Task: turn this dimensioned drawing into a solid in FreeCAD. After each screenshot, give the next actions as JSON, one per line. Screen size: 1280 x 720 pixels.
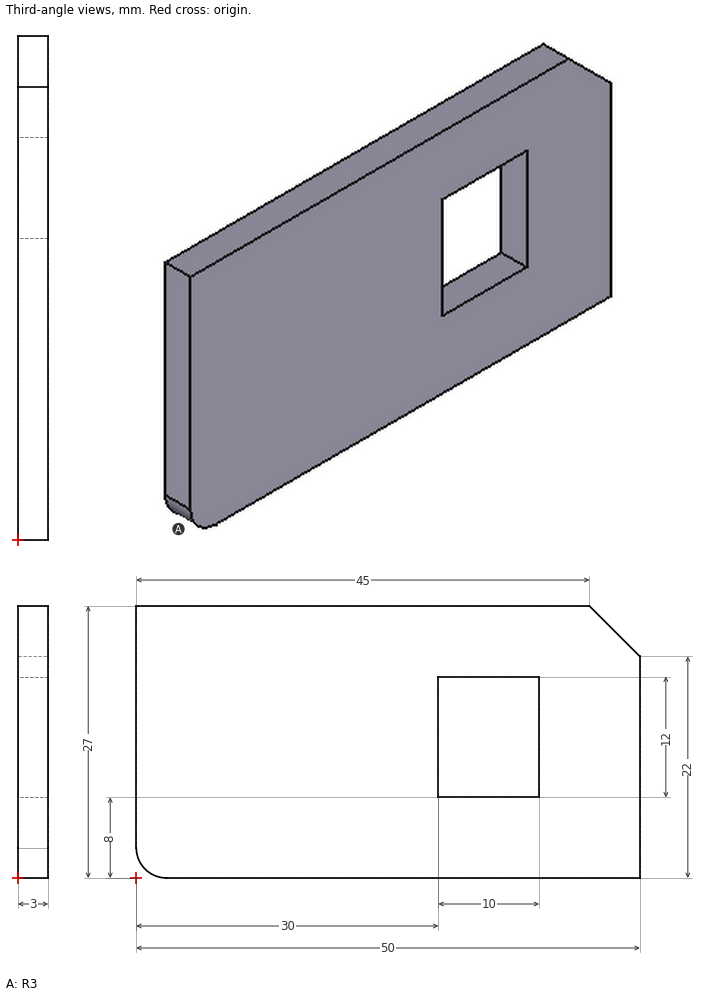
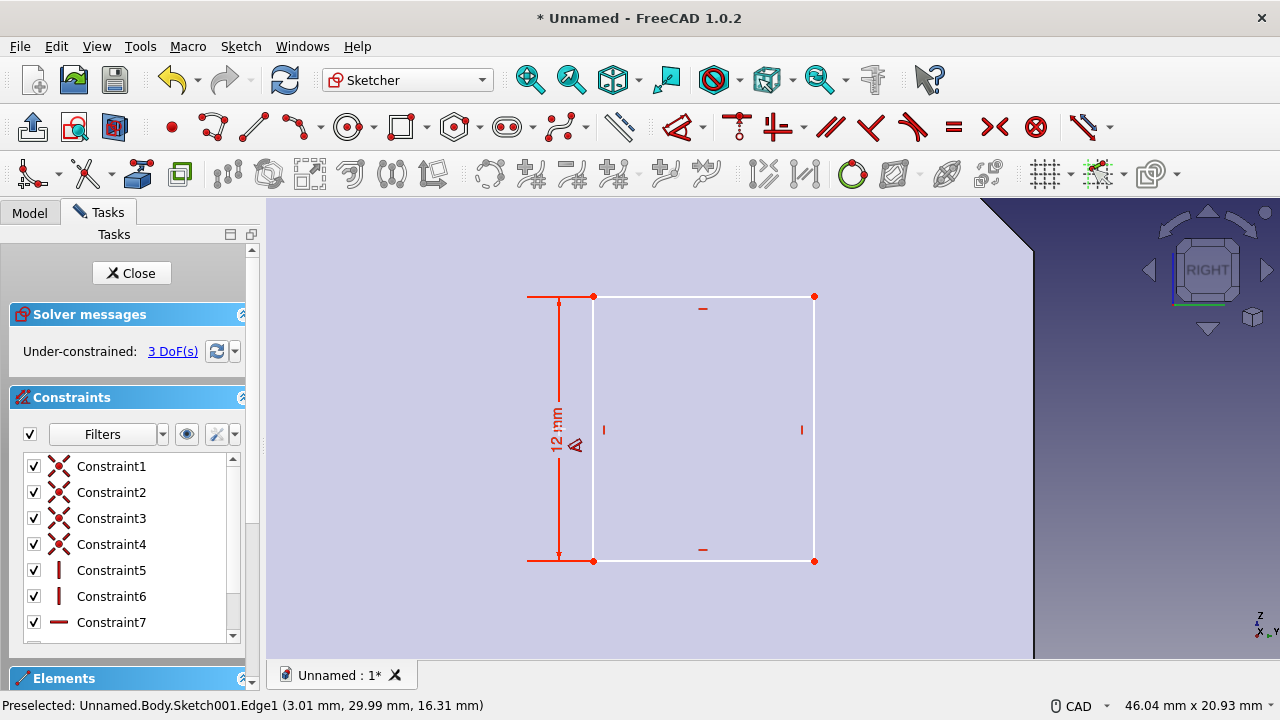
{"action": "left_click", "coordinate": [659, 561]}
{"action": "left_click", "coordinate": [704, 595]}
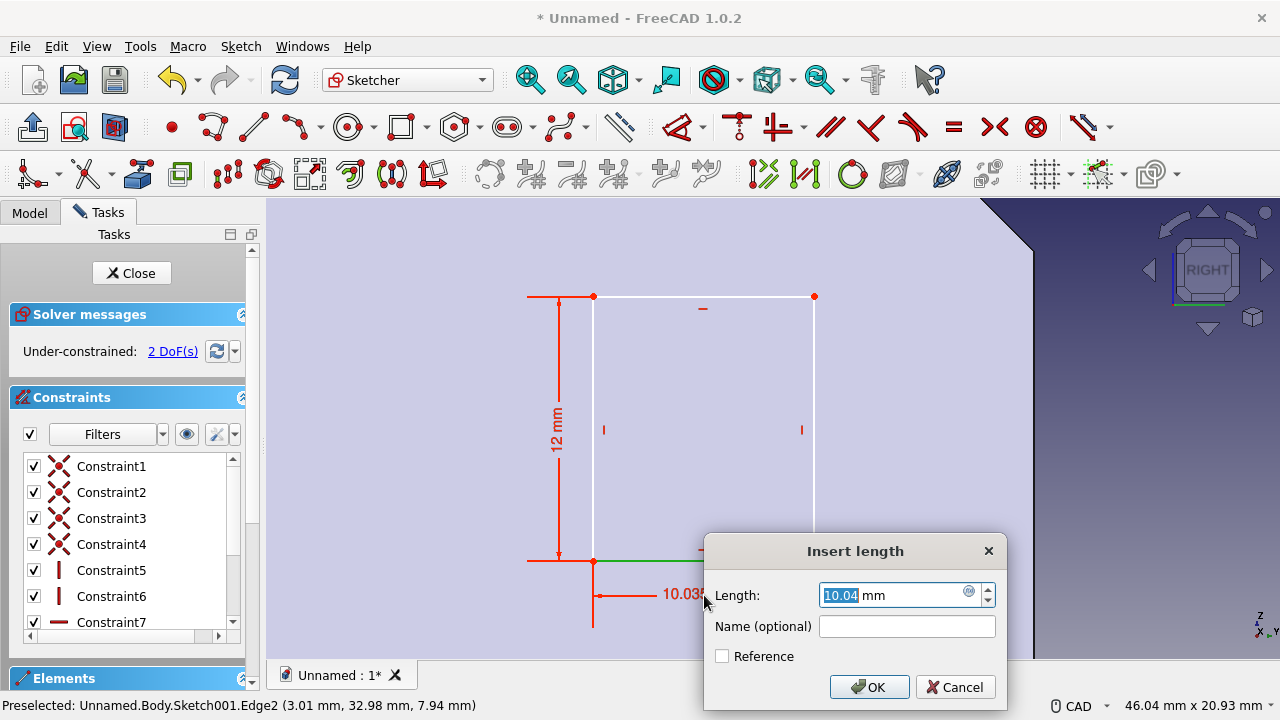
{"action": "type", "text": "10"}
{"action": "key", "text": "Return"}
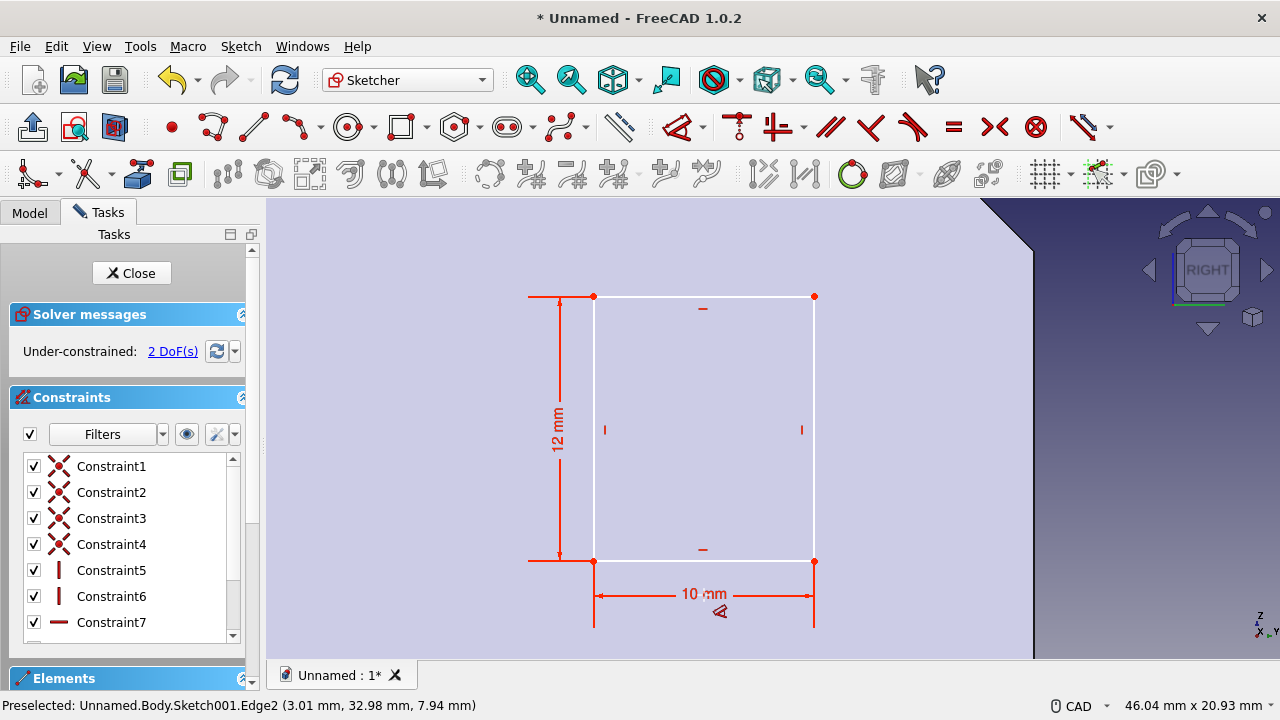
{"action": "left_click", "coordinate": [594, 561]}
{"action": "left_click", "coordinate": [628, 596]}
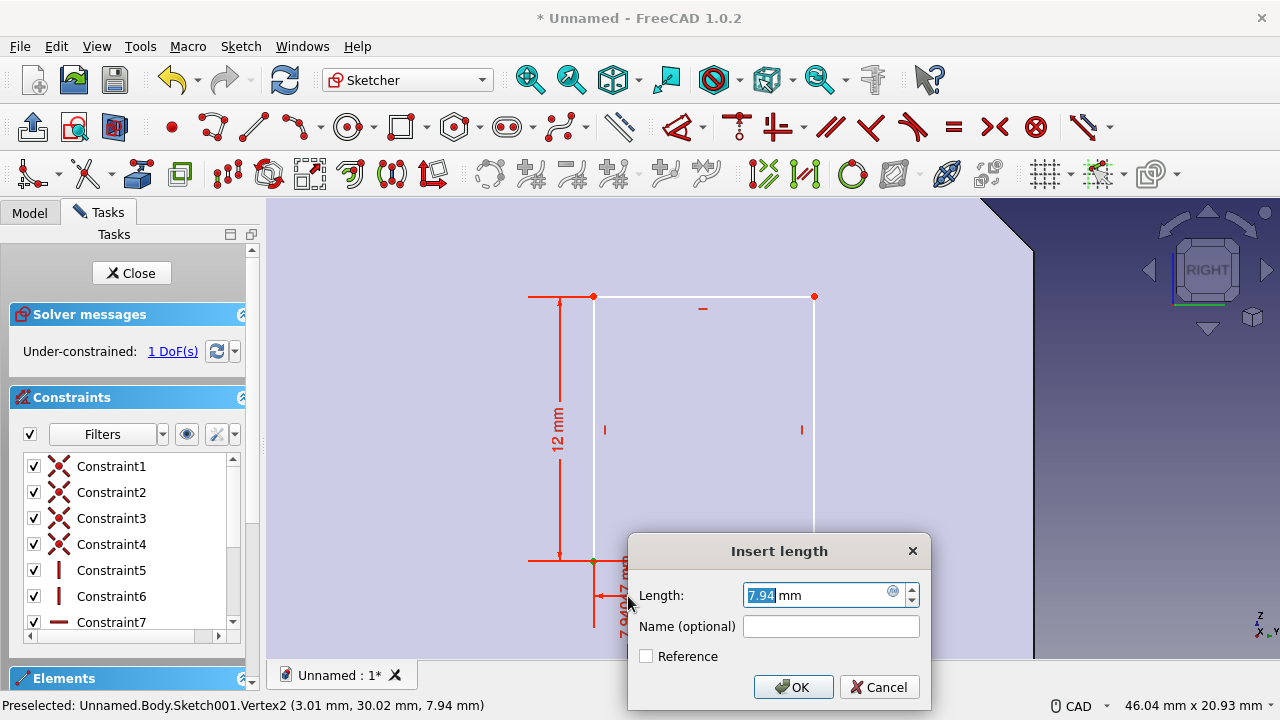
{"action": "type", "text": "8"}
{"action": "key", "text": "Return"}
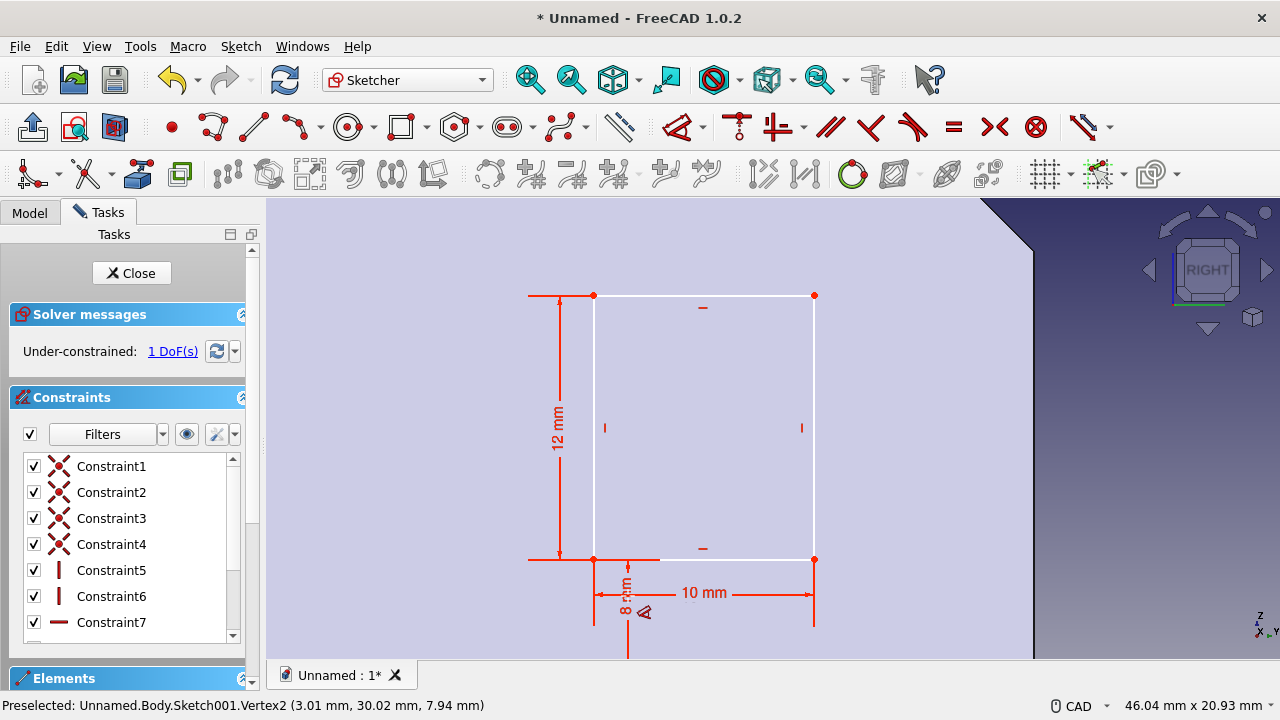
{"action": "left_click", "coordinate": [594, 296]}
{"action": "left_click", "coordinate": [444, 262]}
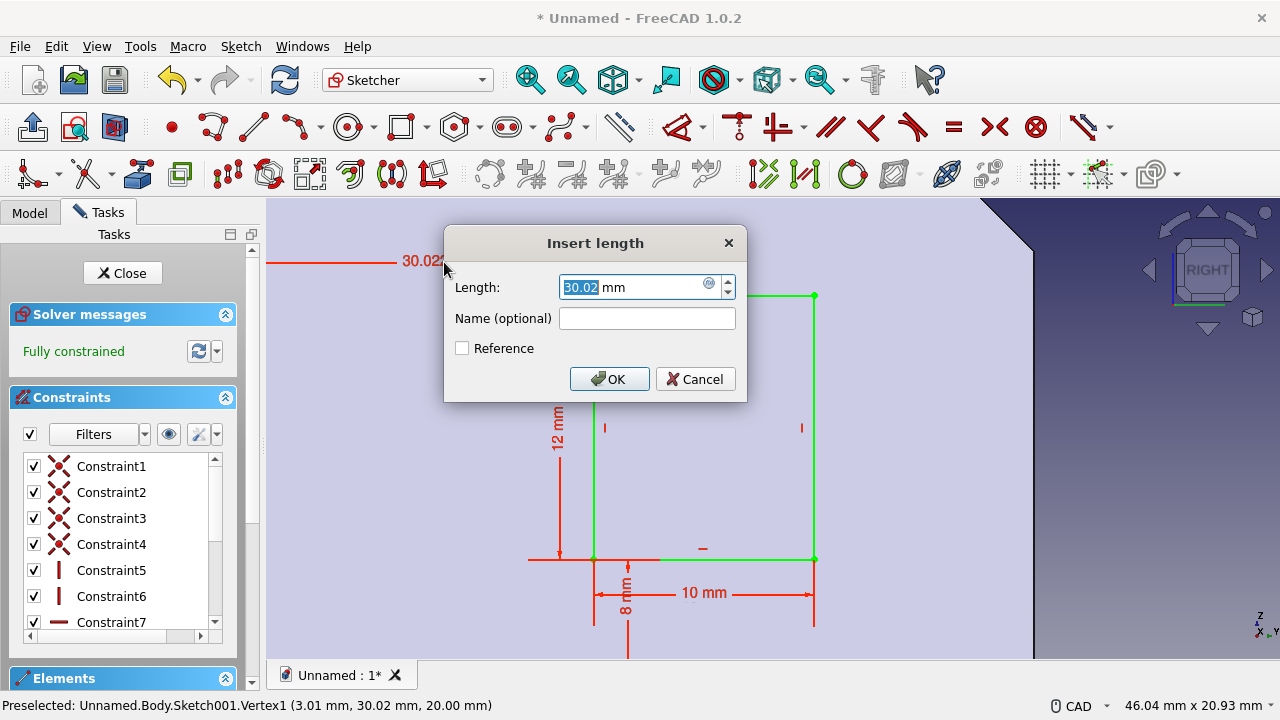
{"action": "type", "text": "30"}
{"action": "key", "text": "Return"}
{"action": "key", "text": "Escape"}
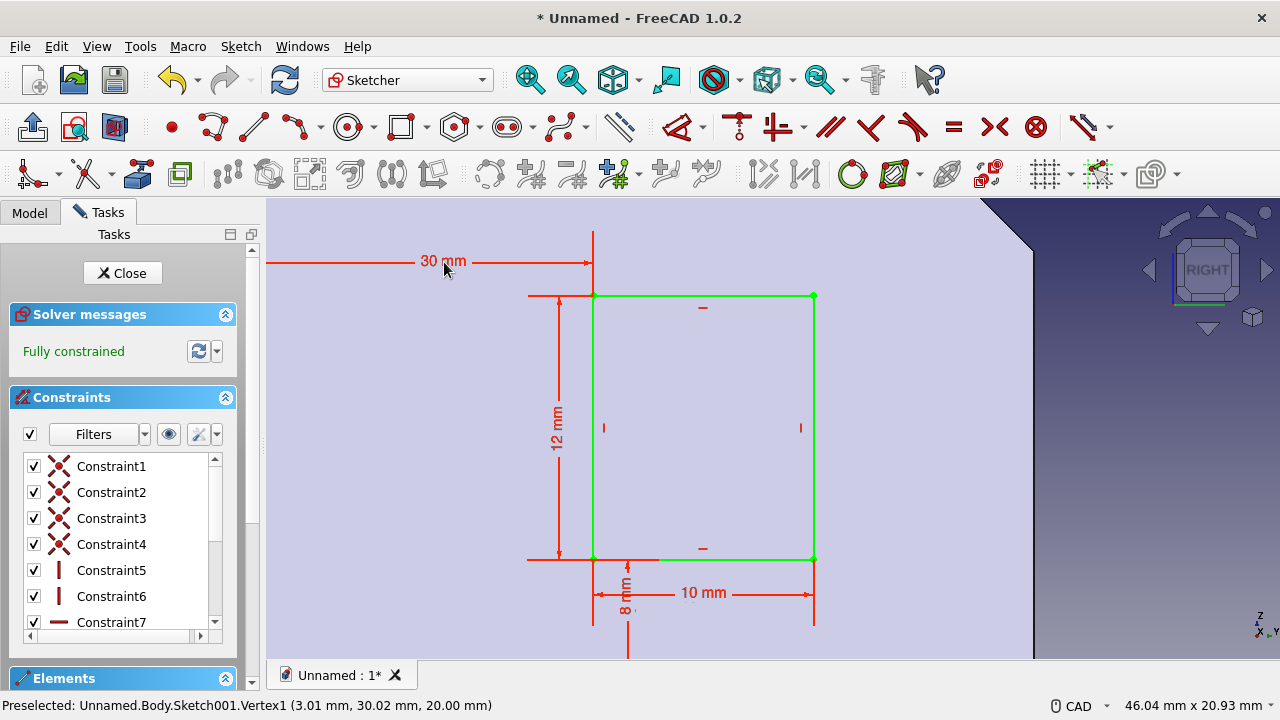
{"action": "left_click", "coordinate": [123, 273]}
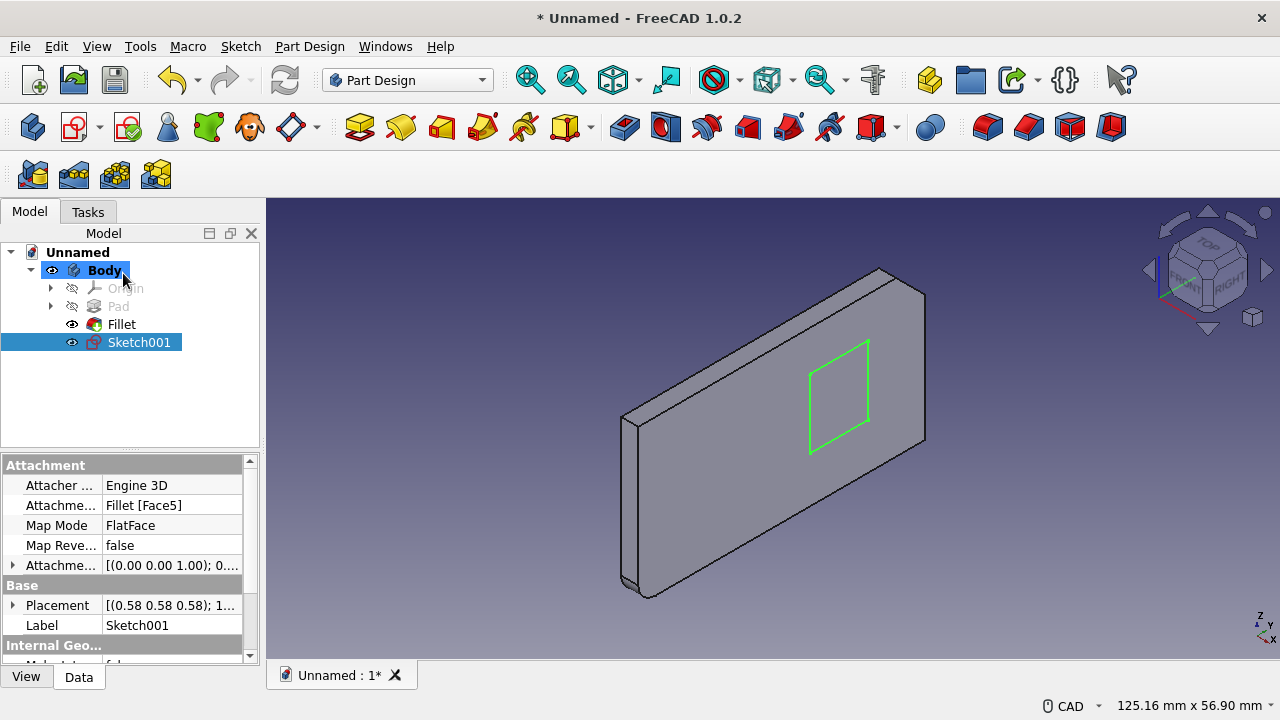
{"action": "left_click", "coordinate": [625, 128]}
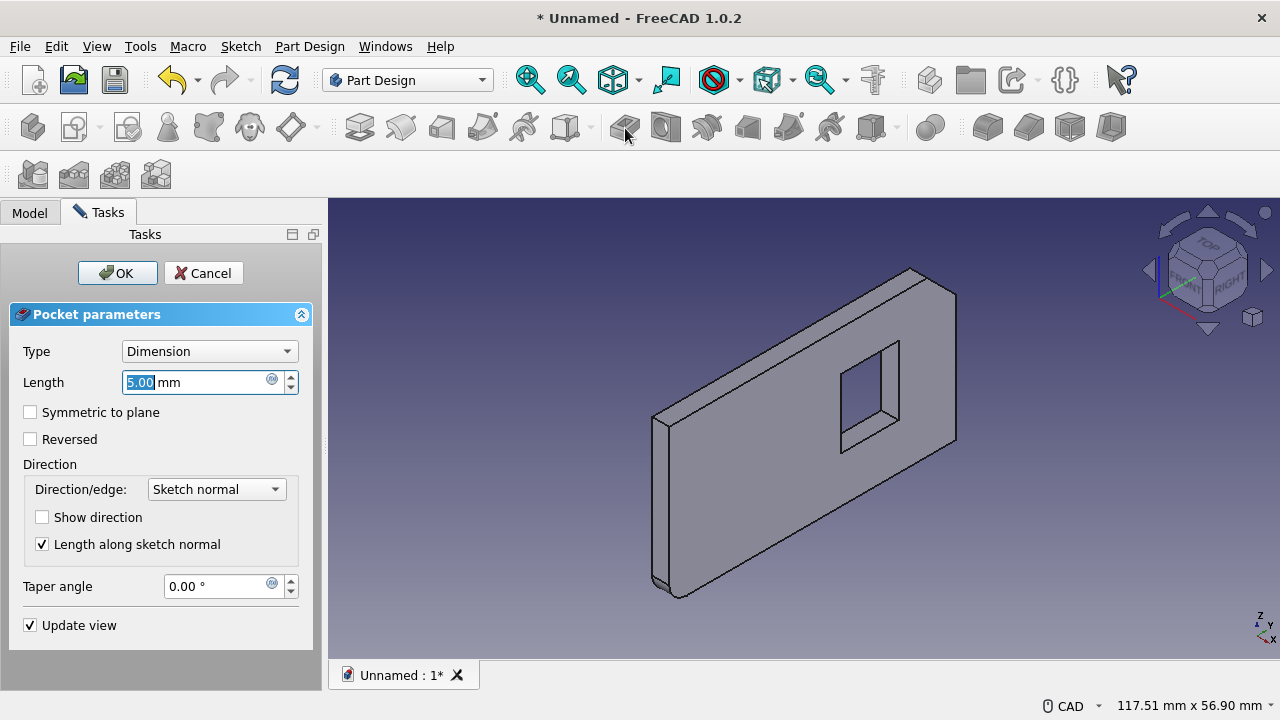
{"action": "left_click", "coordinate": [210, 352]}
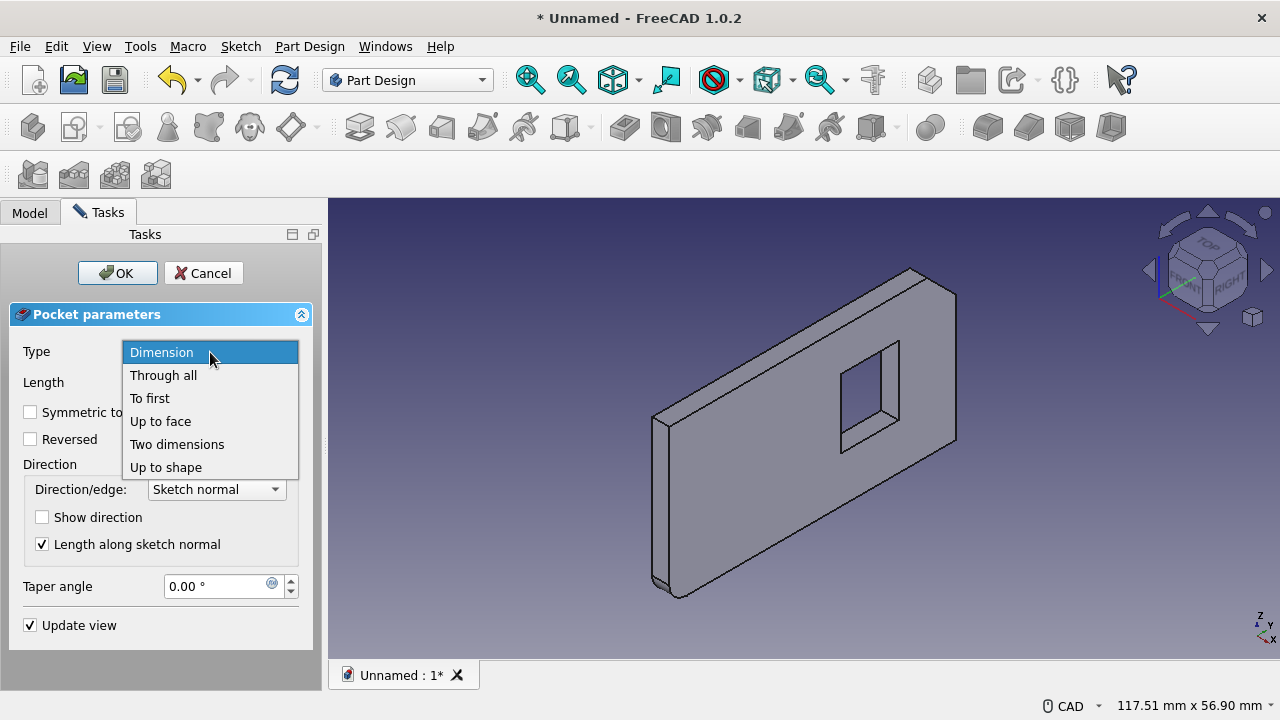
{"action": "left_click", "coordinate": [208, 376]}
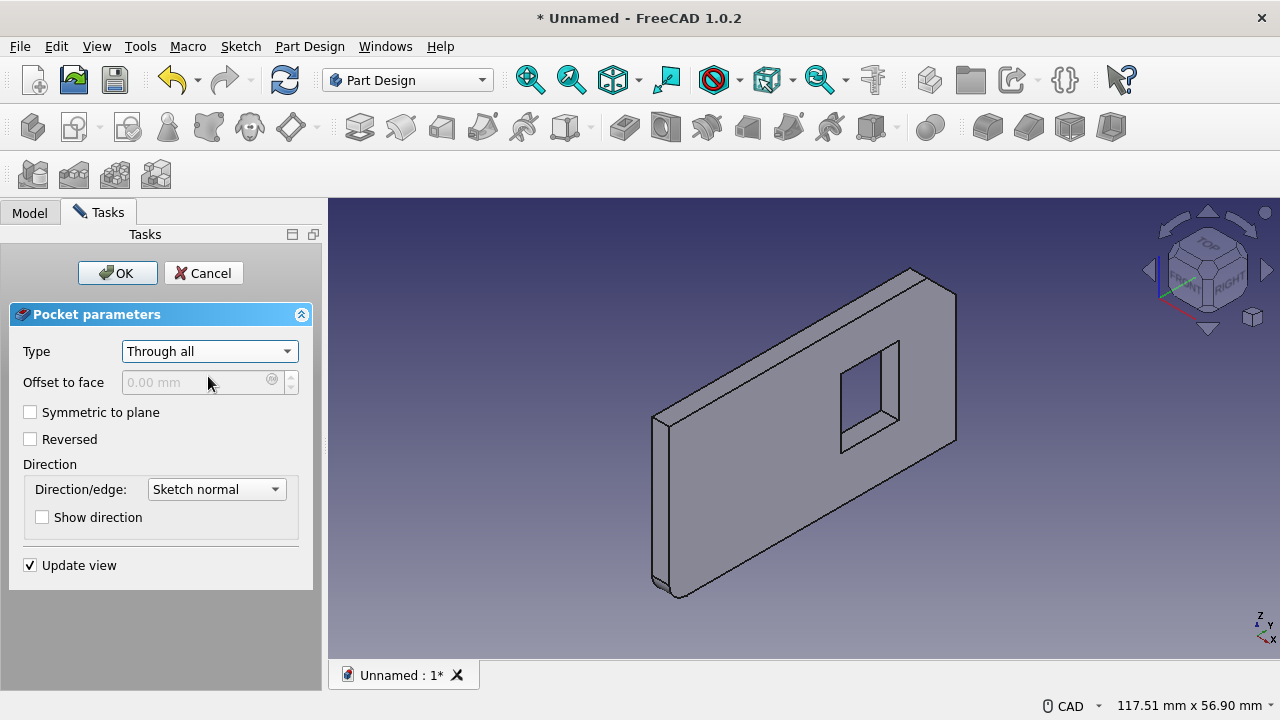
{"action": "left_click", "coordinate": [118, 273]}